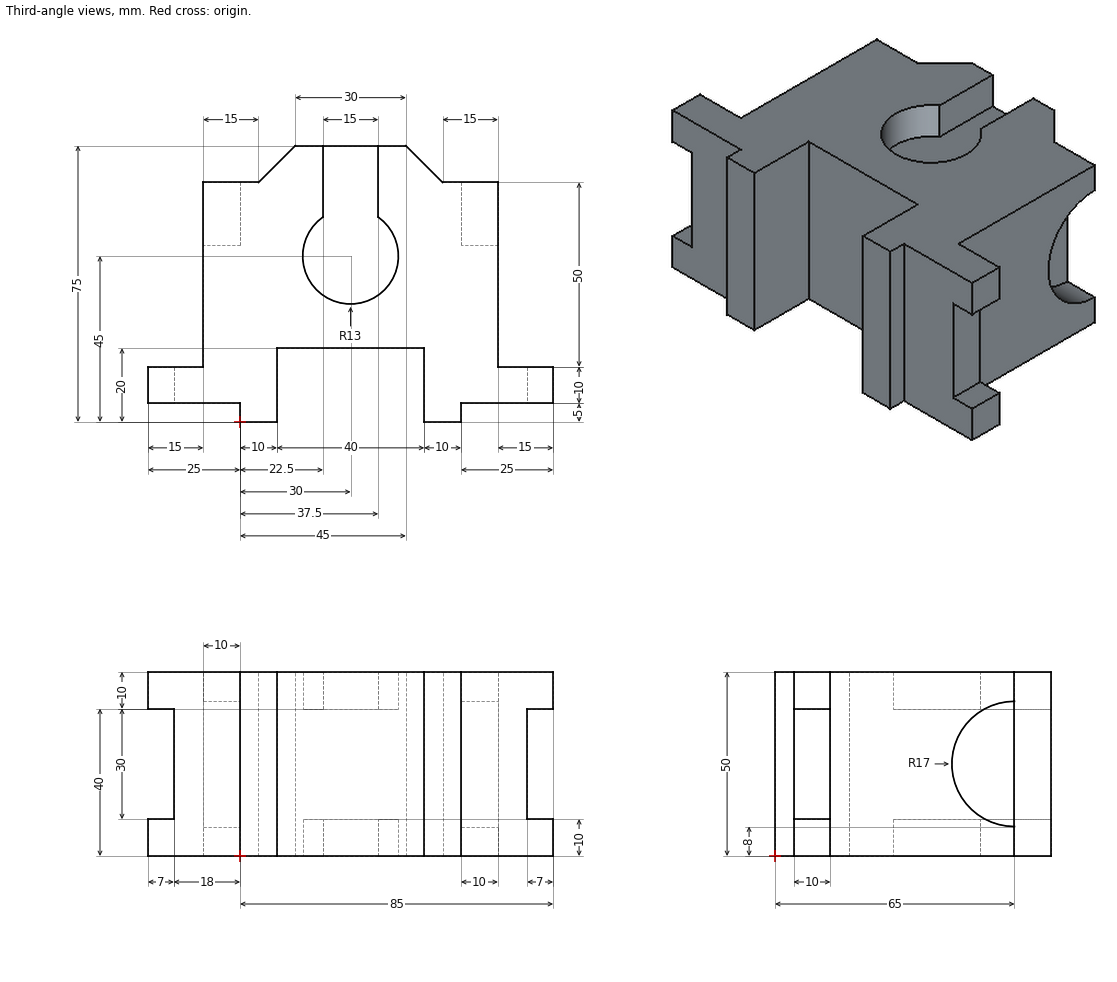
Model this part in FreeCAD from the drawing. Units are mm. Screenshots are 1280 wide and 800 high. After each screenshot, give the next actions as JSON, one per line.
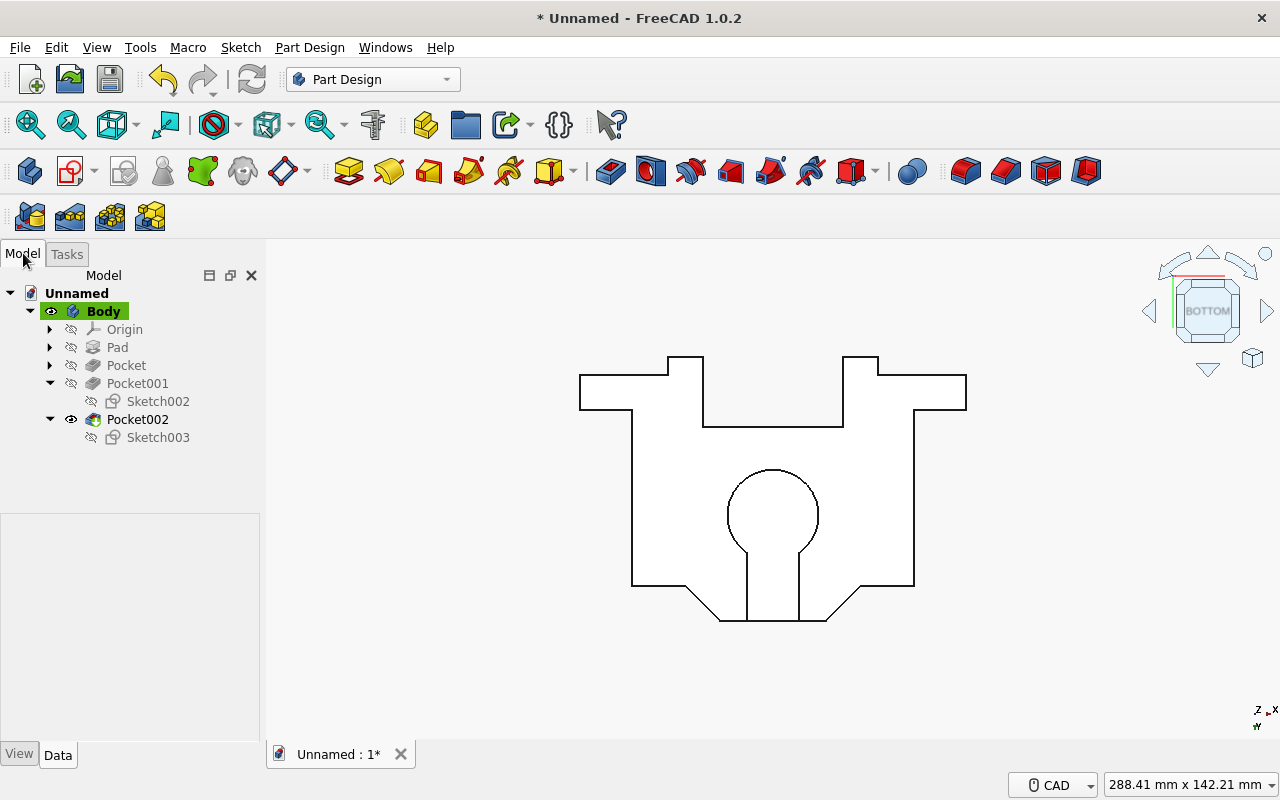
{"action": "left_click", "coordinate": [50, 329]}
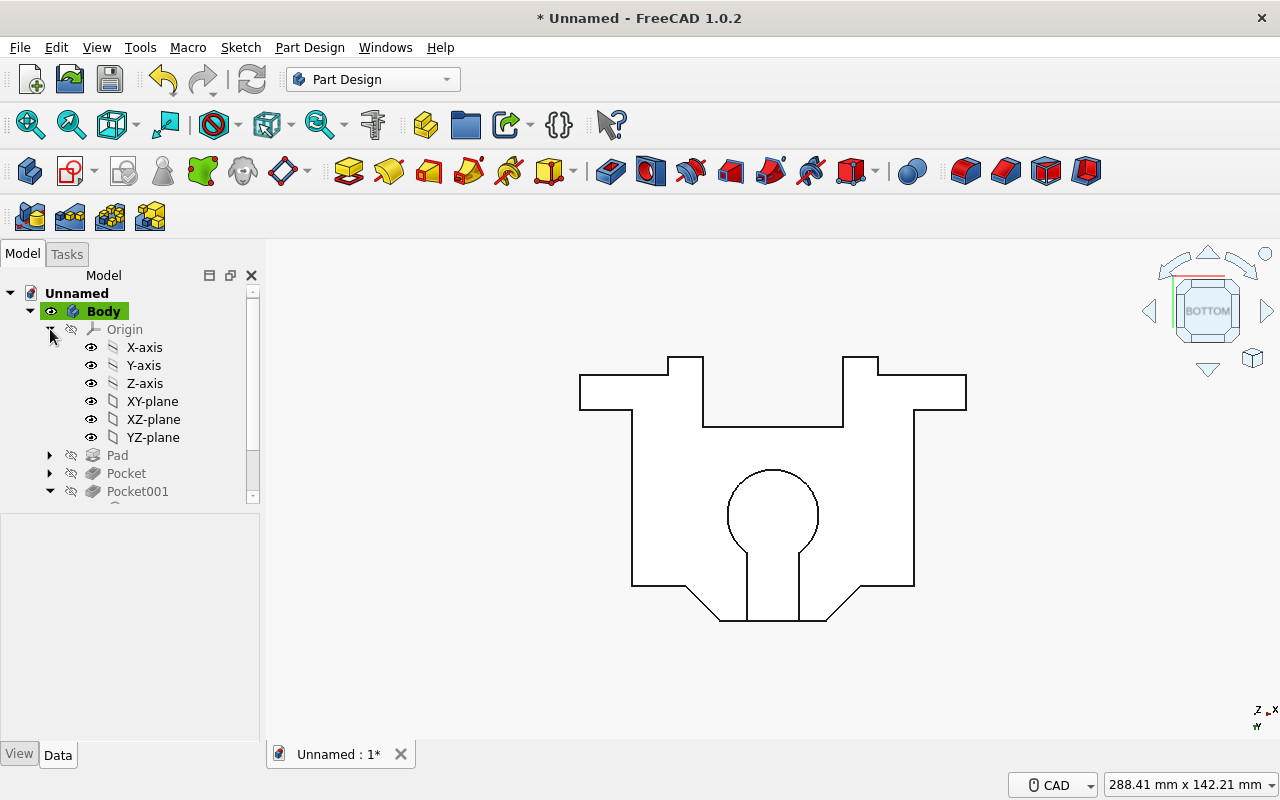
{"action": "left_click", "coordinate": [136, 401]}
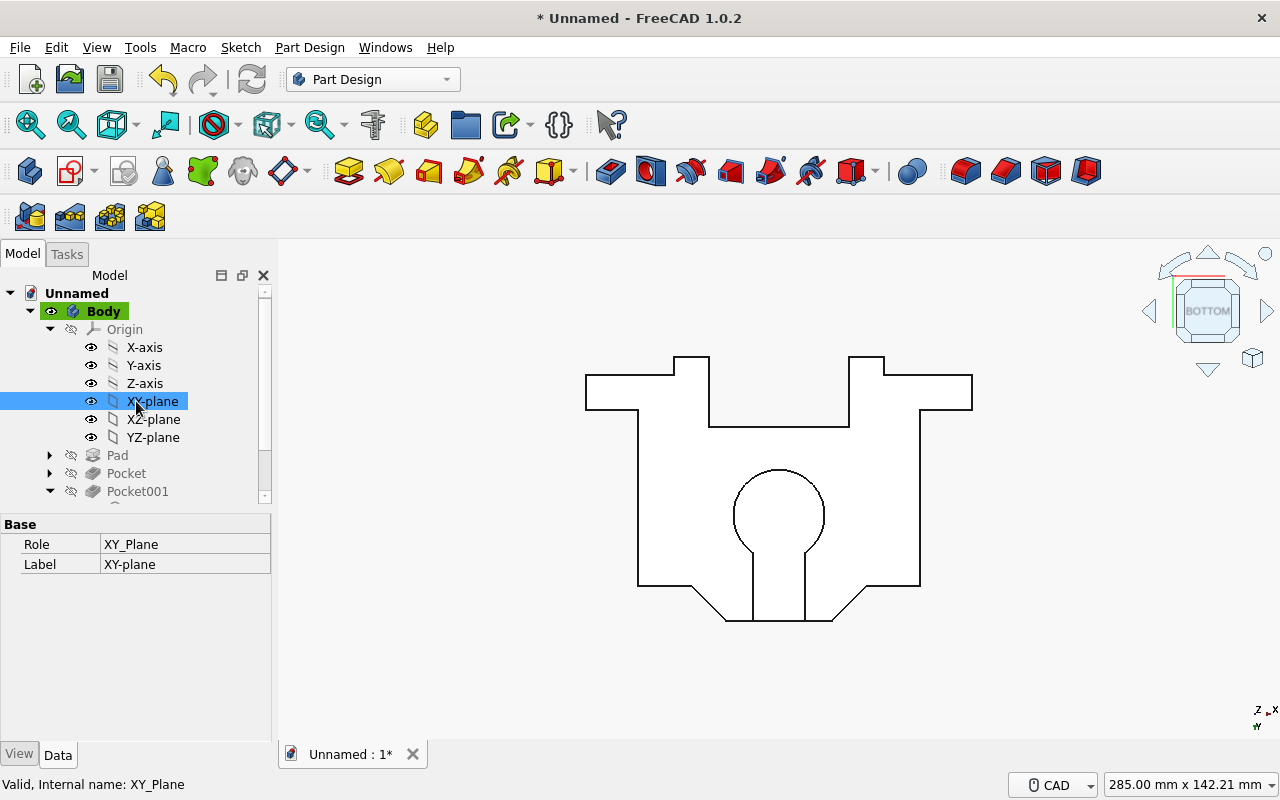
{"action": "left_click", "coordinate": [284, 172]}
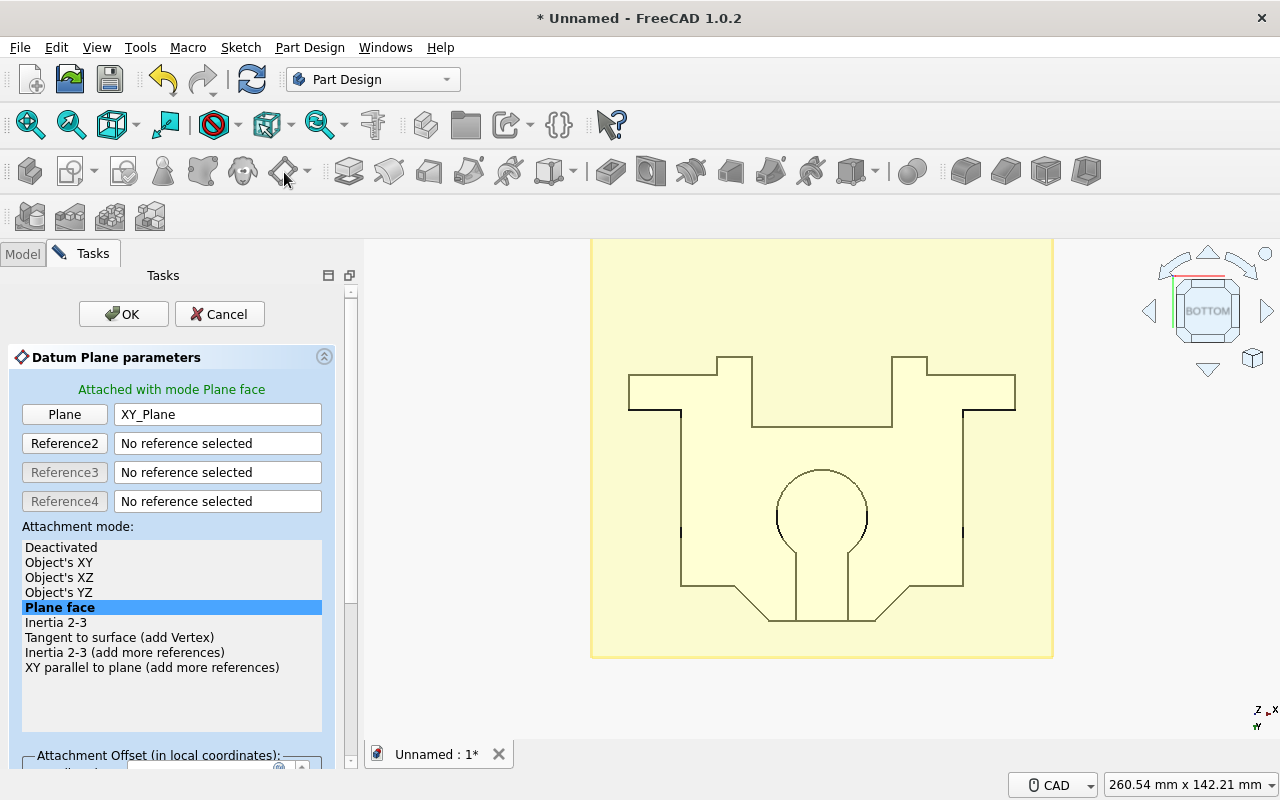
{"action": "scroll", "coordinate": [351, 526], "scroll_direction": "down", "scroll_amount": 3}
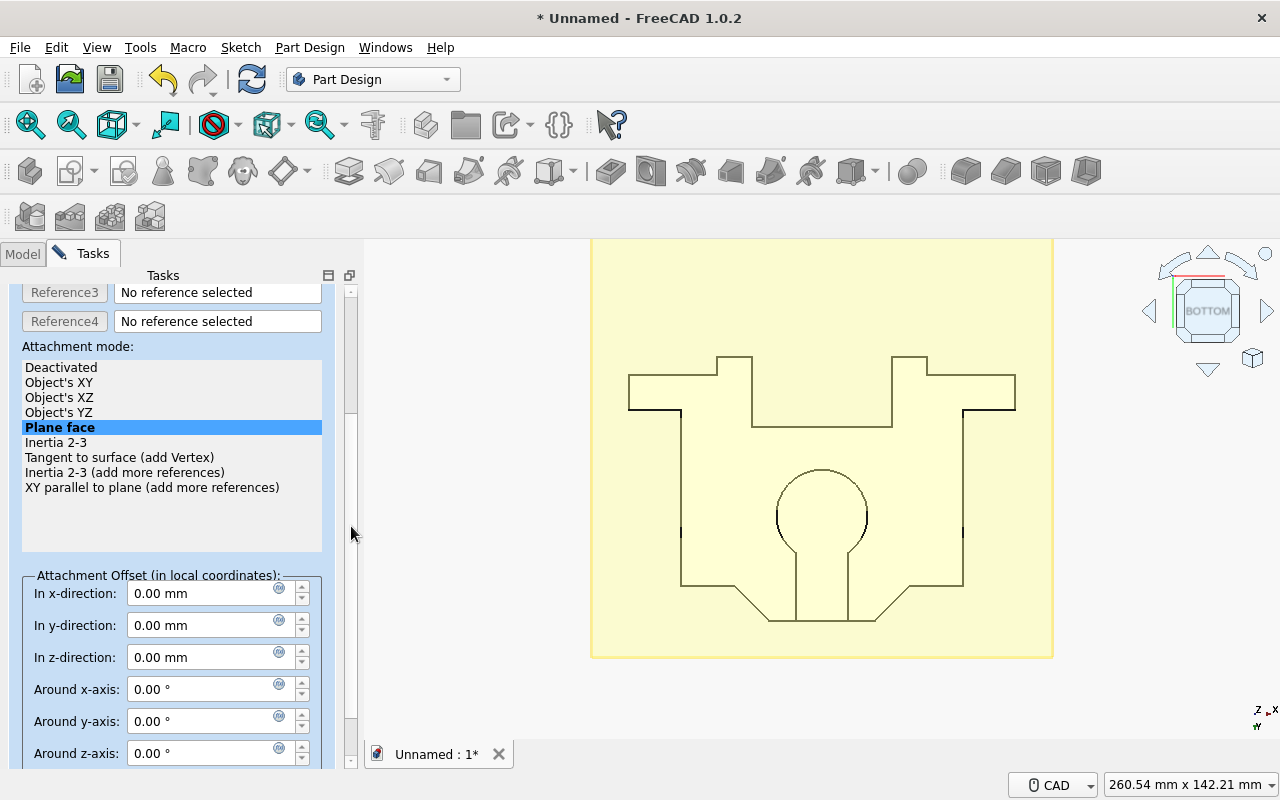
{"action": "triple_click", "coordinate": [210, 657]}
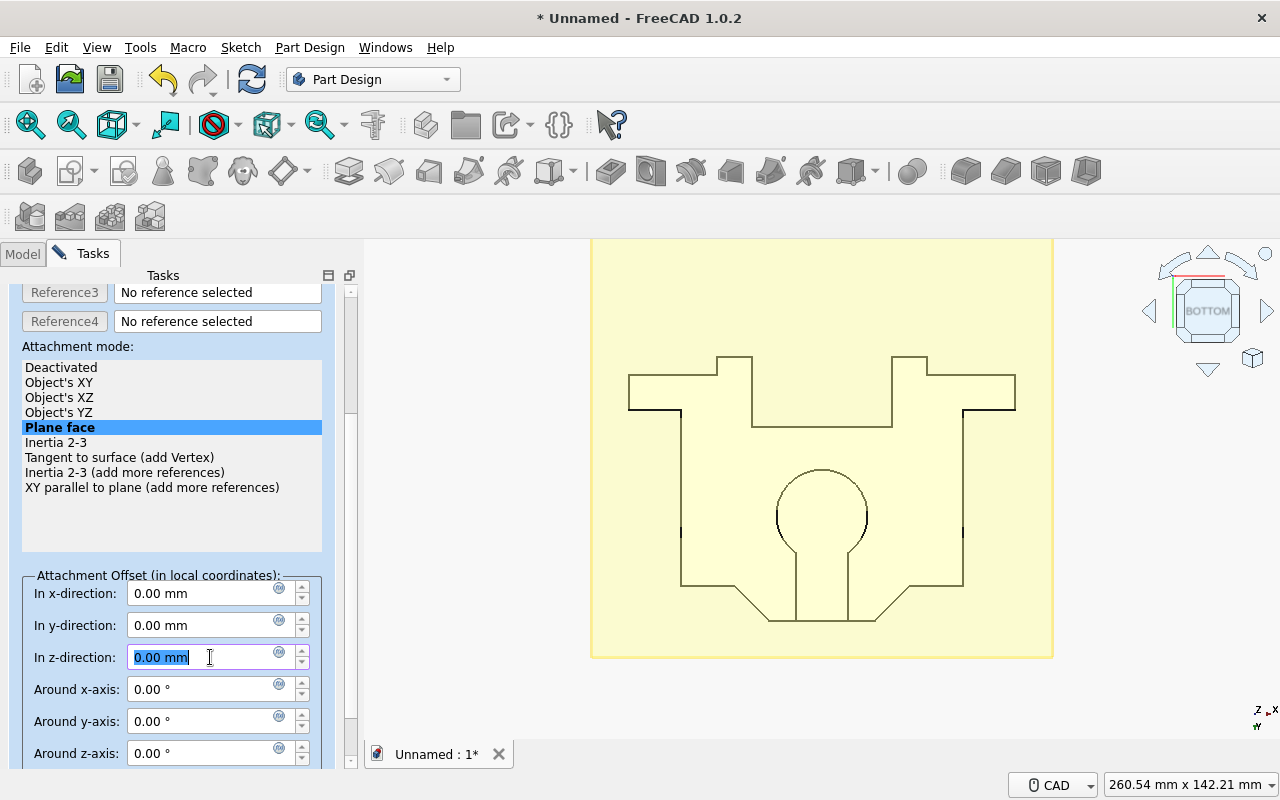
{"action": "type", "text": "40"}
{"action": "key", "text": "Tab"}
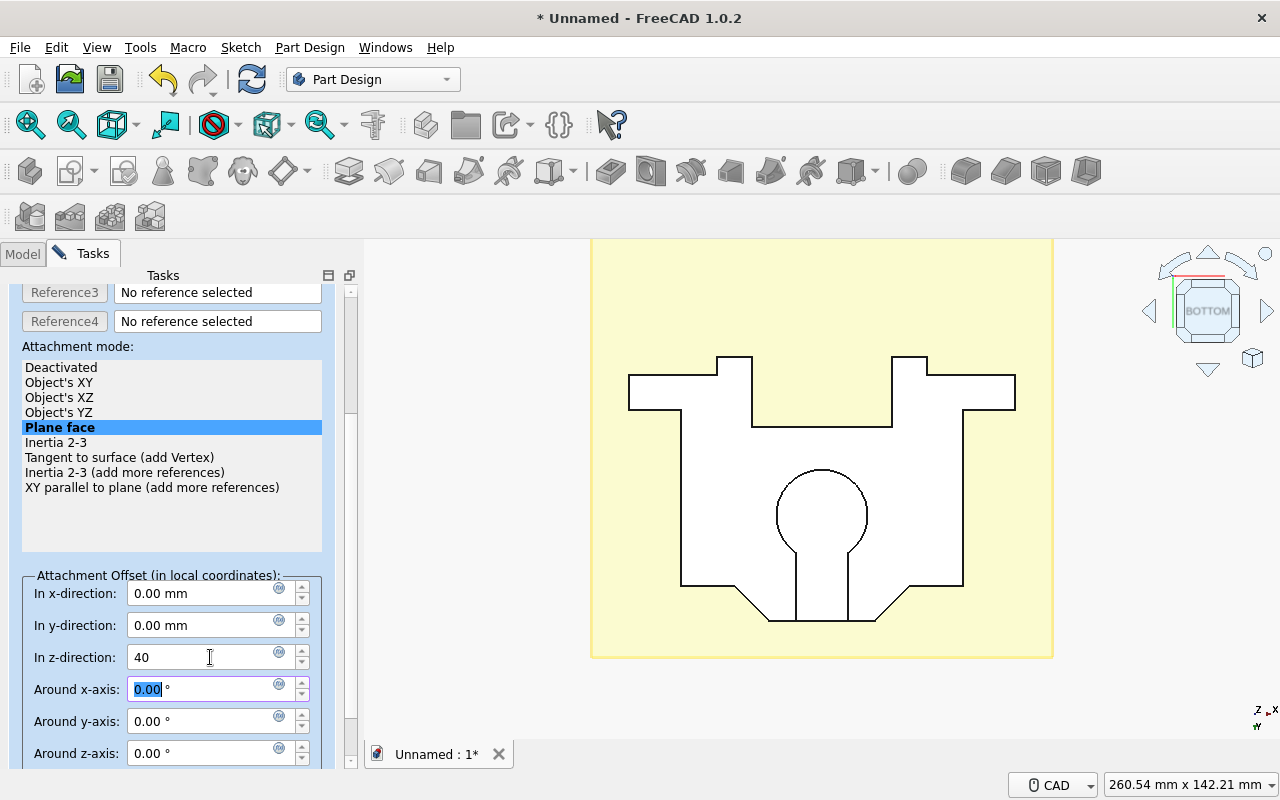
{"action": "scroll", "coordinate": [351, 526], "scroll_direction": "up", "scroll_amount": 4}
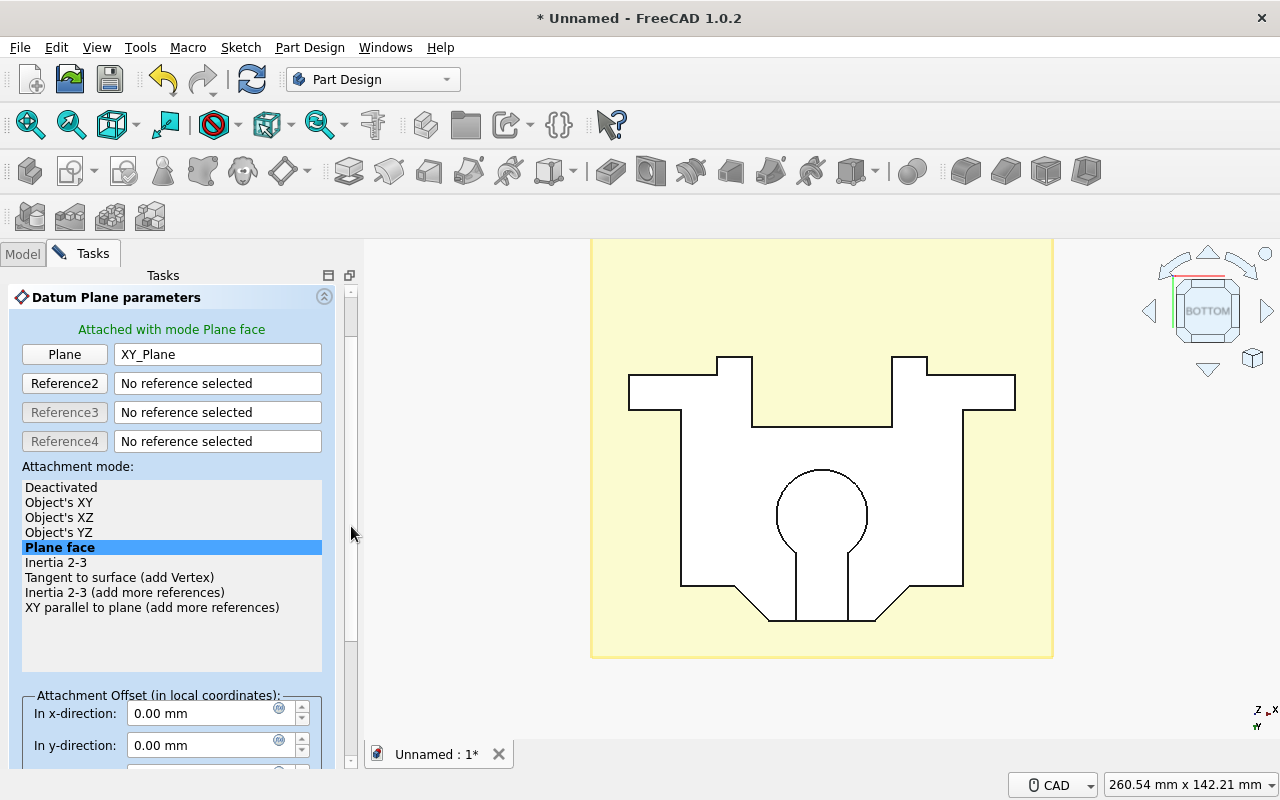
{"action": "left_click", "coordinate": [124, 314]}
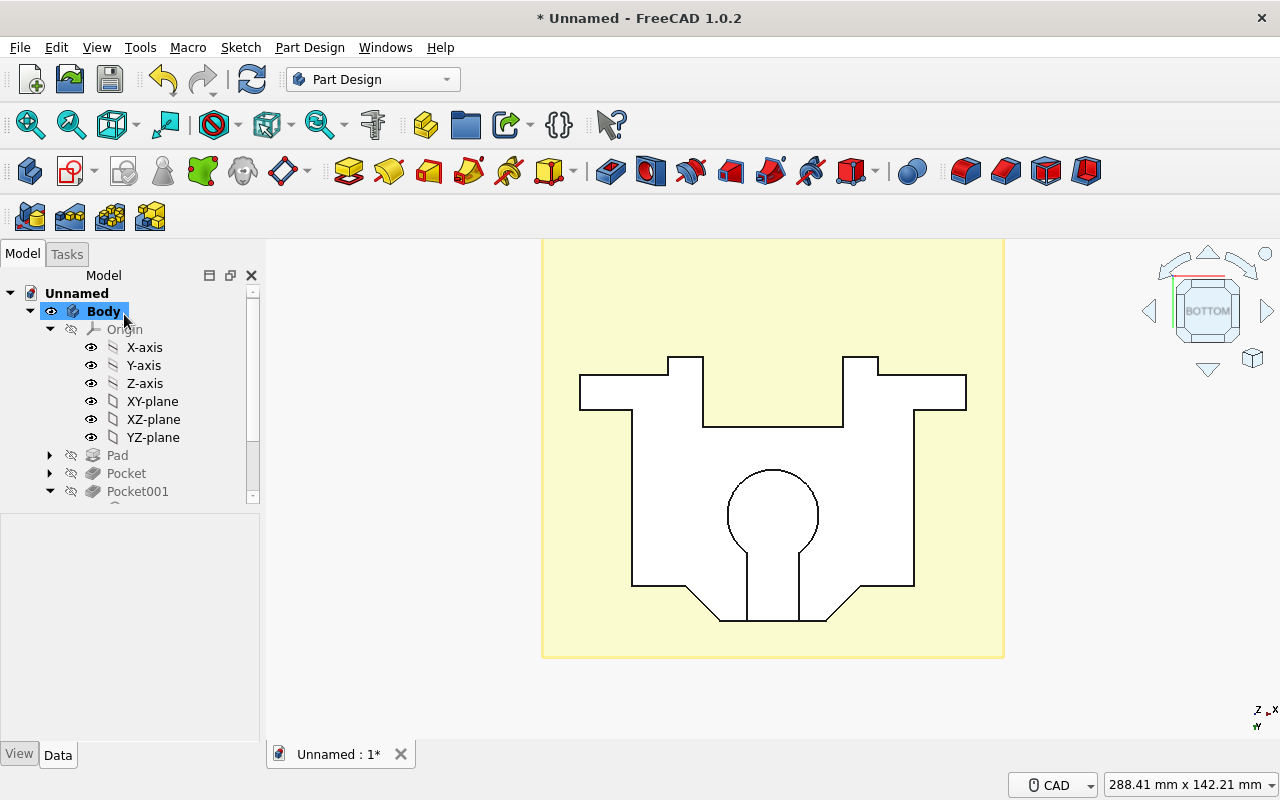
{"action": "scroll", "coordinate": [100, 397], "scroll_direction": "down", "scroll_amount": 3}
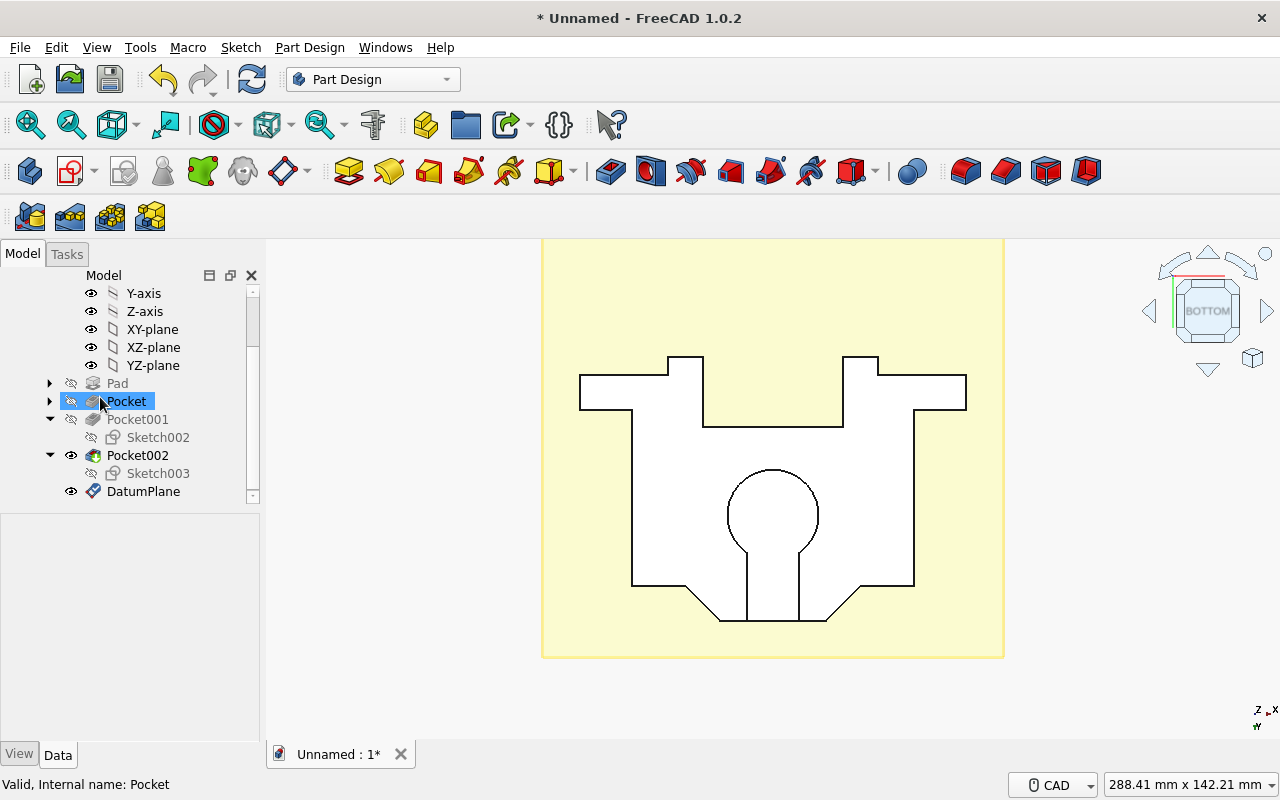
{"action": "left_click", "coordinate": [116, 491]}